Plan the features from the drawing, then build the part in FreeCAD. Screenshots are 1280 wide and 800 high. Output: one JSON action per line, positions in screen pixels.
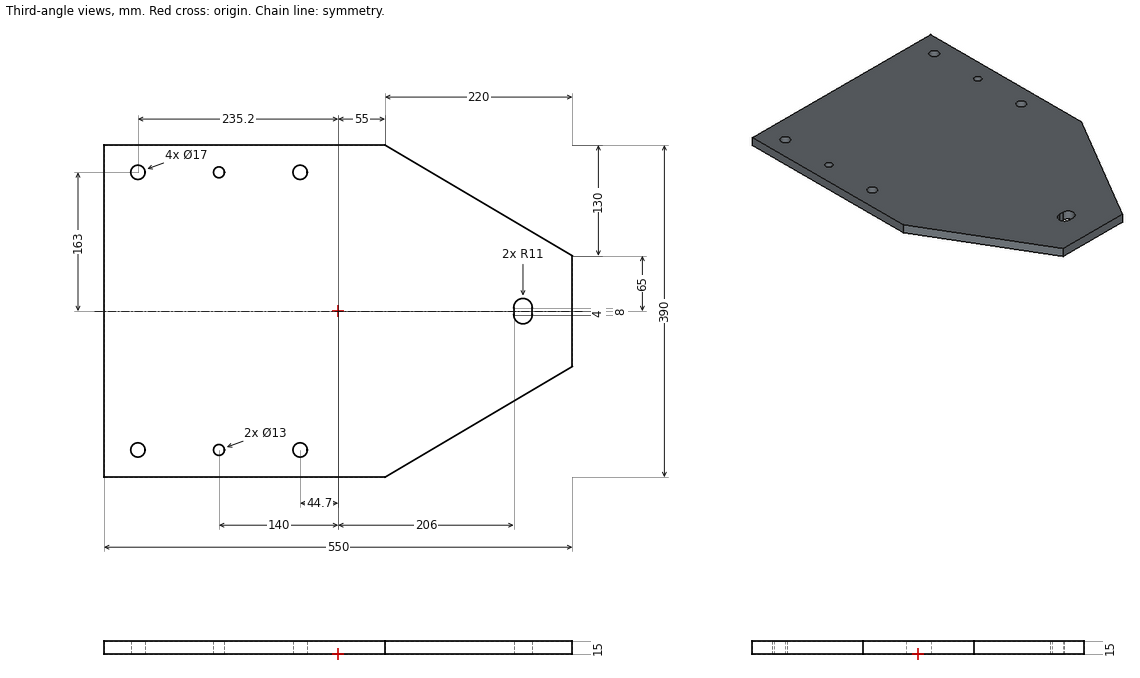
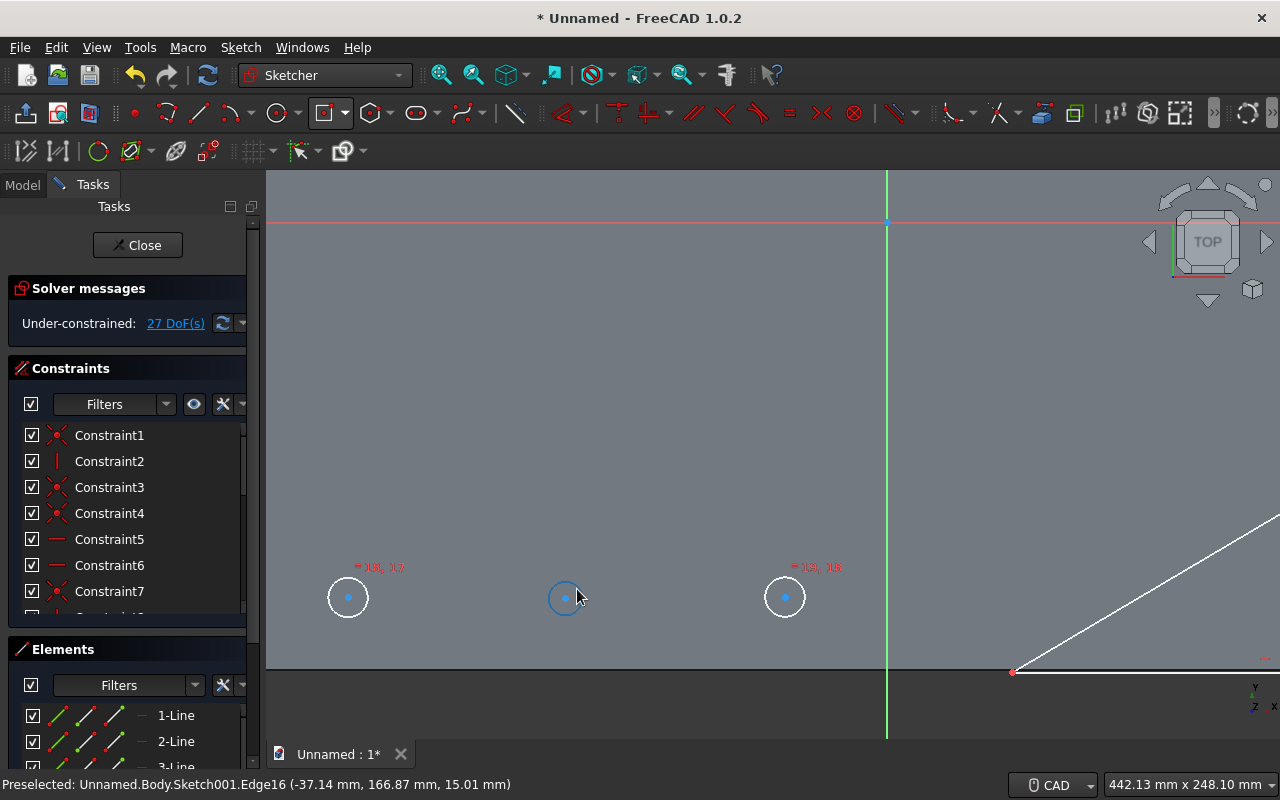
{"action": "left_click", "coordinate": [577, 587]}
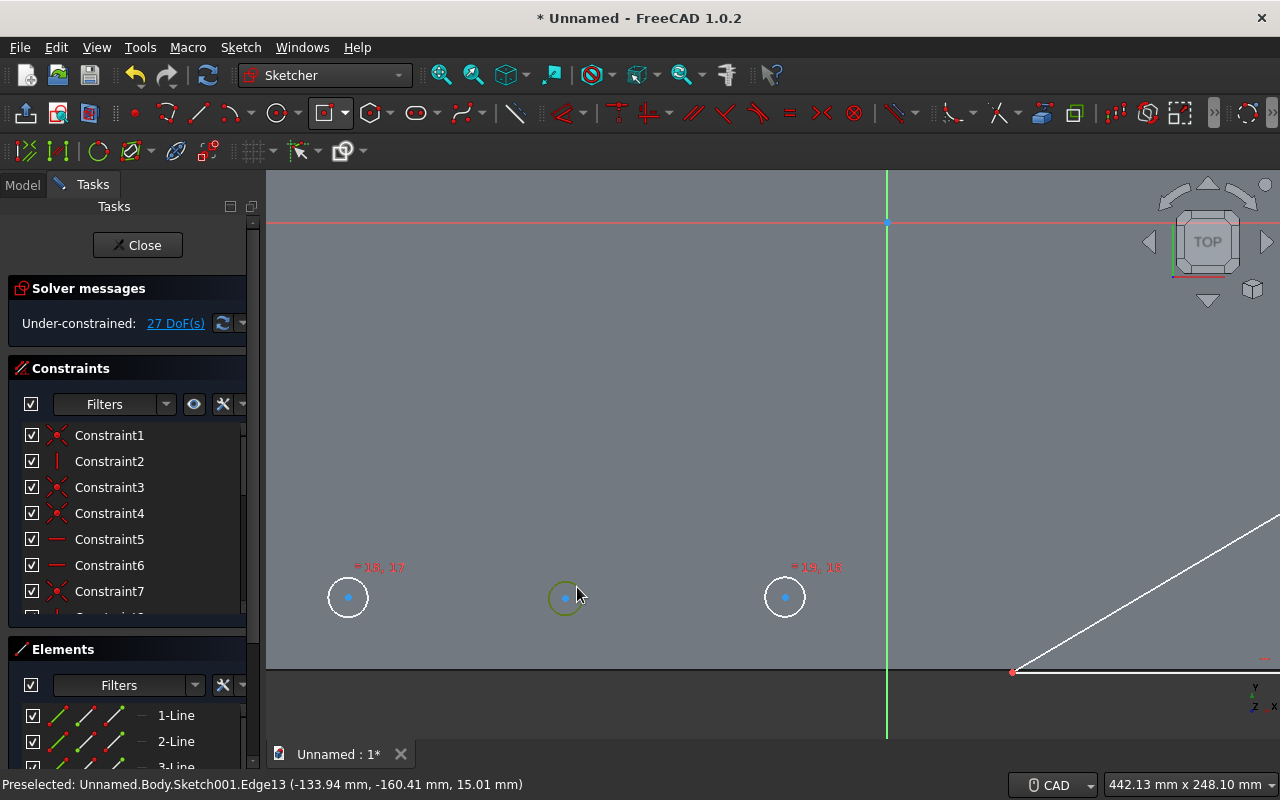
{"action": "scroll", "coordinate": [577, 589], "scroll_direction": "down", "scroll_amount": 5}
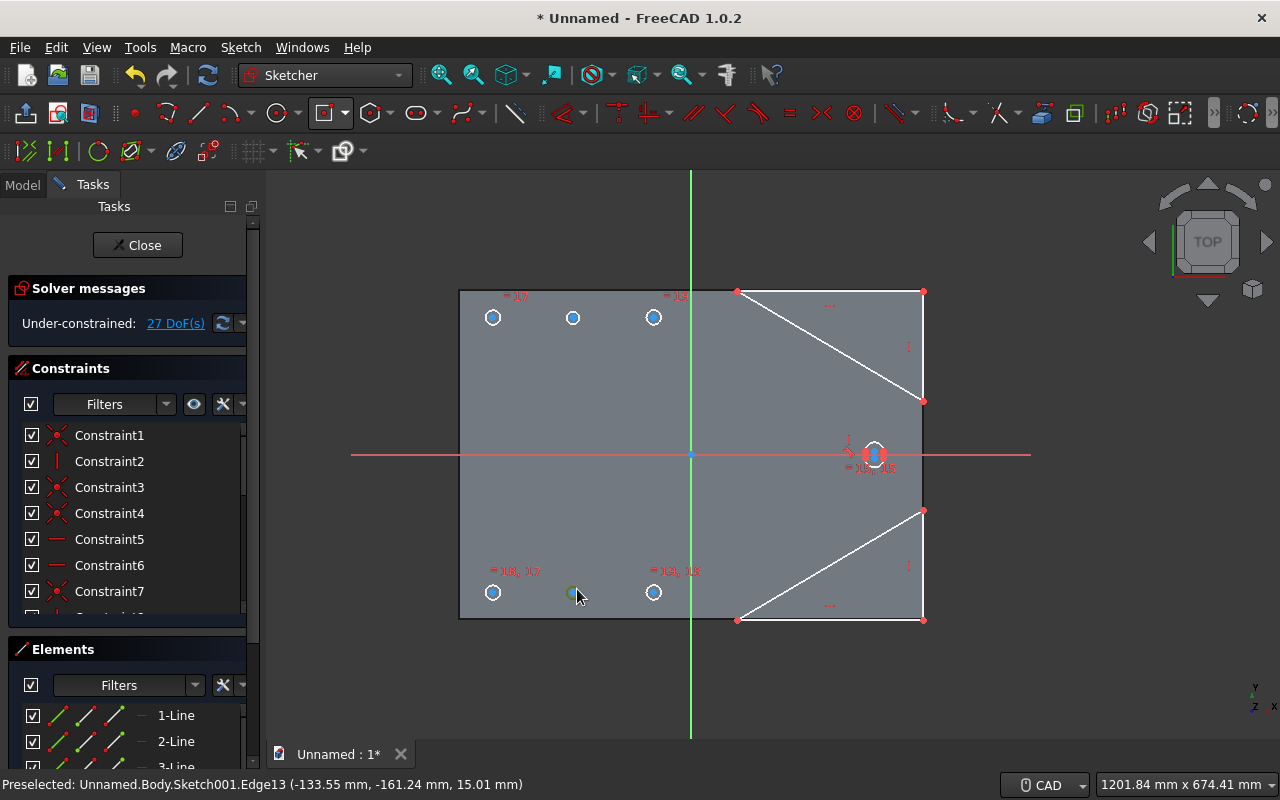
{"action": "scroll", "coordinate": [577, 314], "scroll_direction": "up", "scroll_amount": 5}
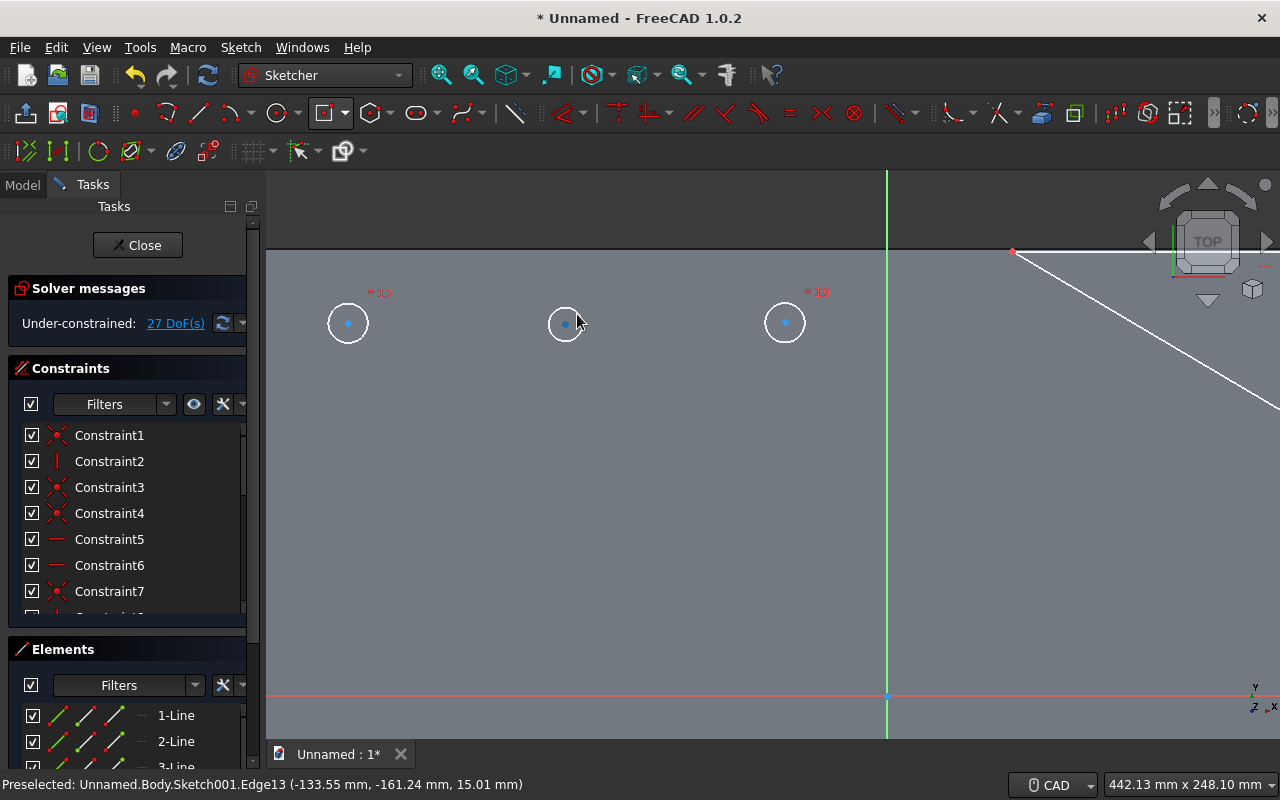
{"action": "left_click", "coordinate": [577, 313]}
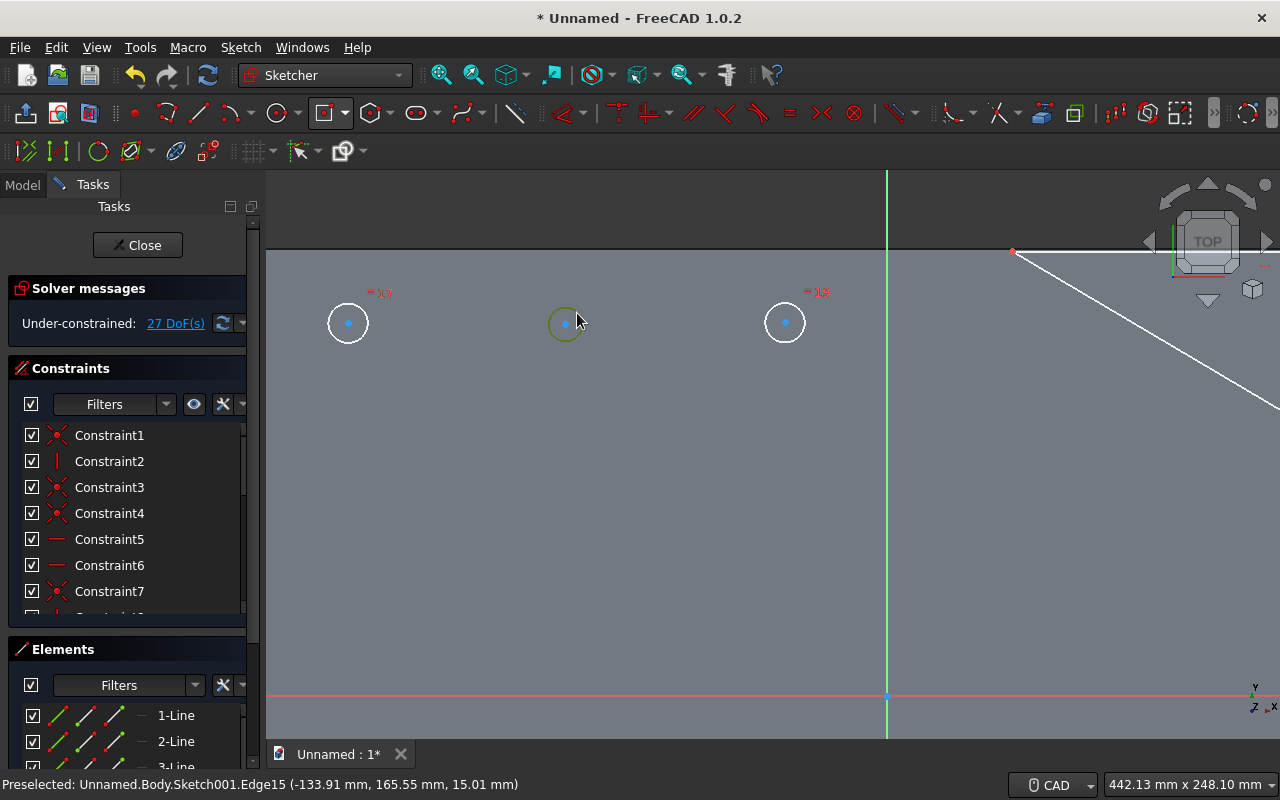
{"action": "left_click", "coordinate": [790, 114]}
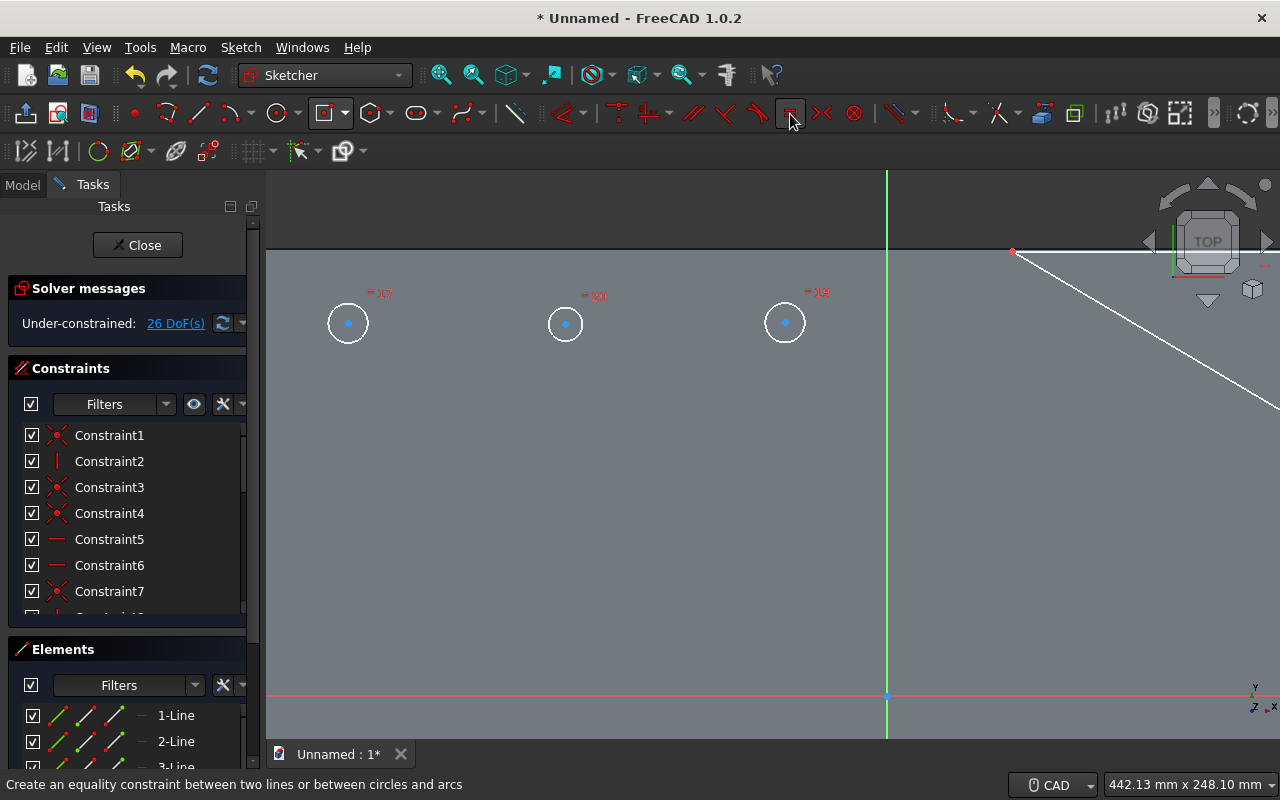
{"action": "left_click", "coordinate": [348, 323]}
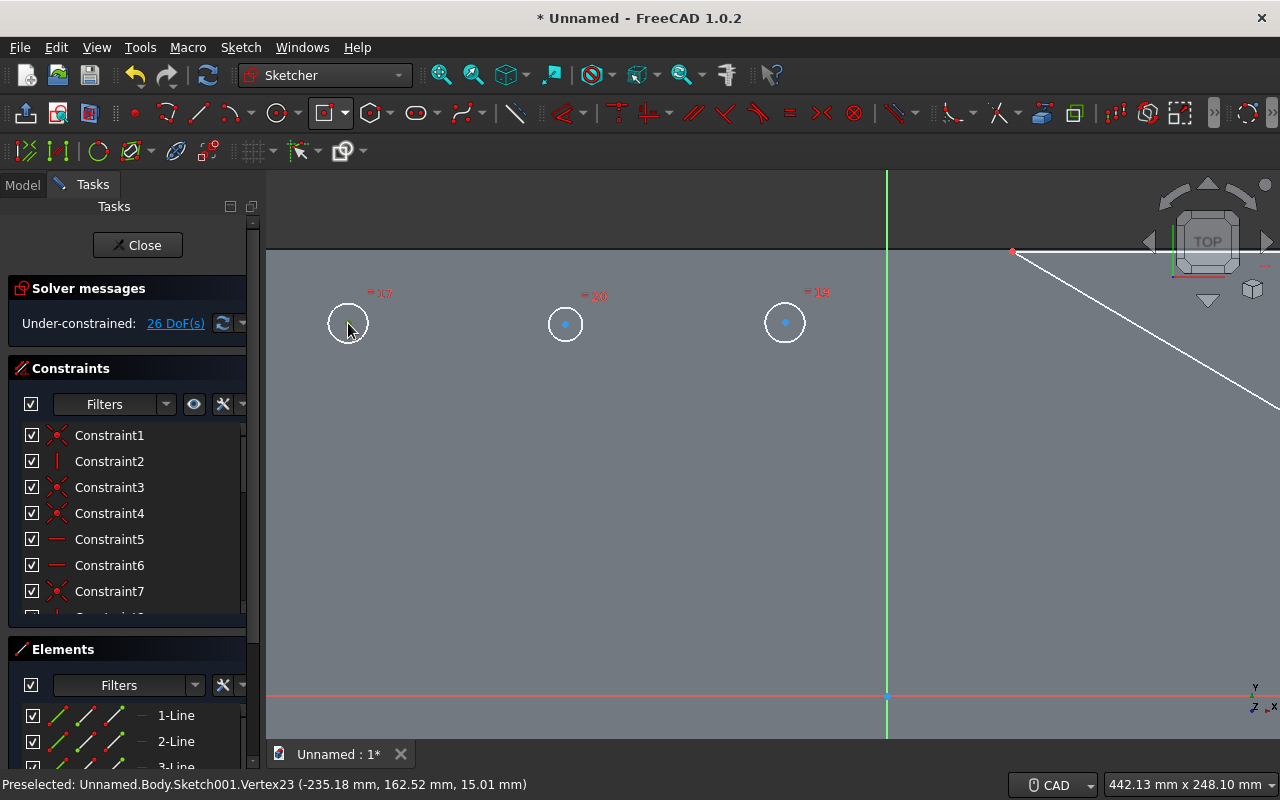
{"action": "scroll", "coordinate": [577, 314], "scroll_direction": "down", "scroll_amount": 5}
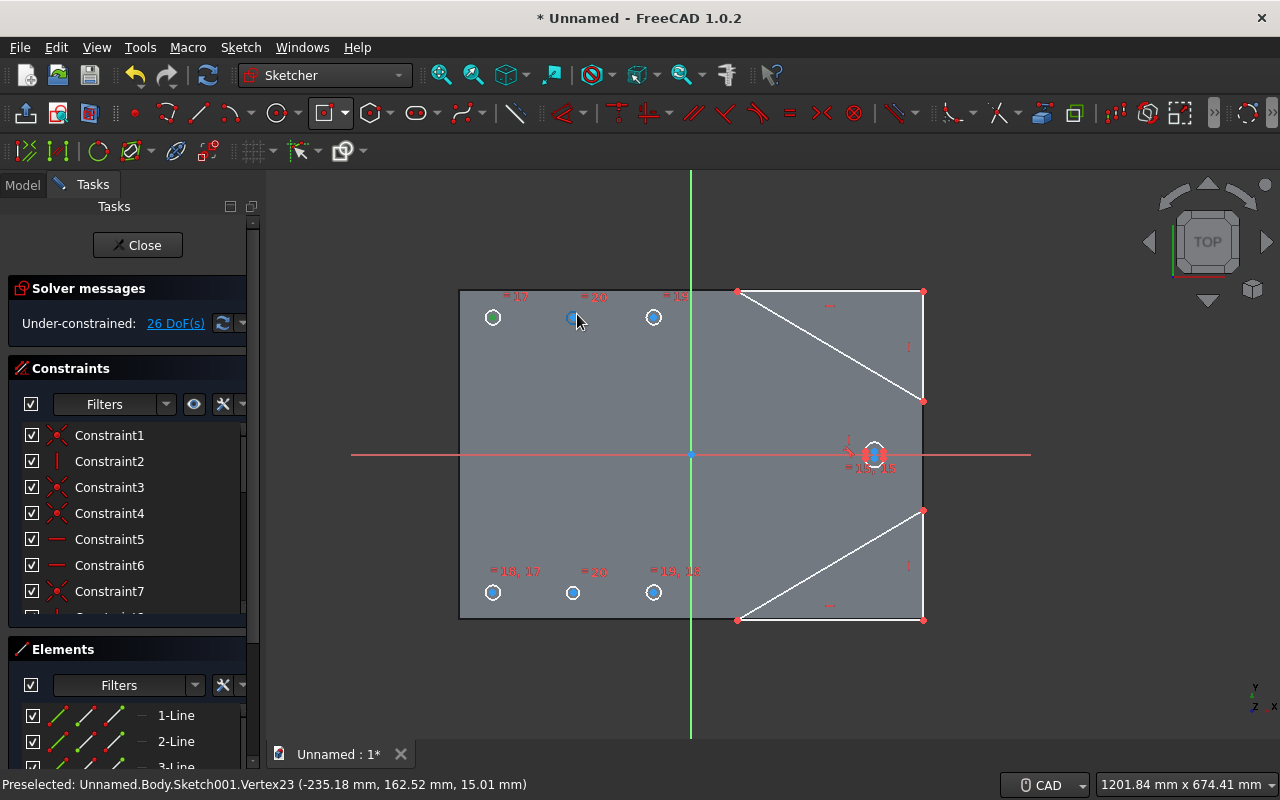
{"action": "left_click", "coordinate": [493, 593]}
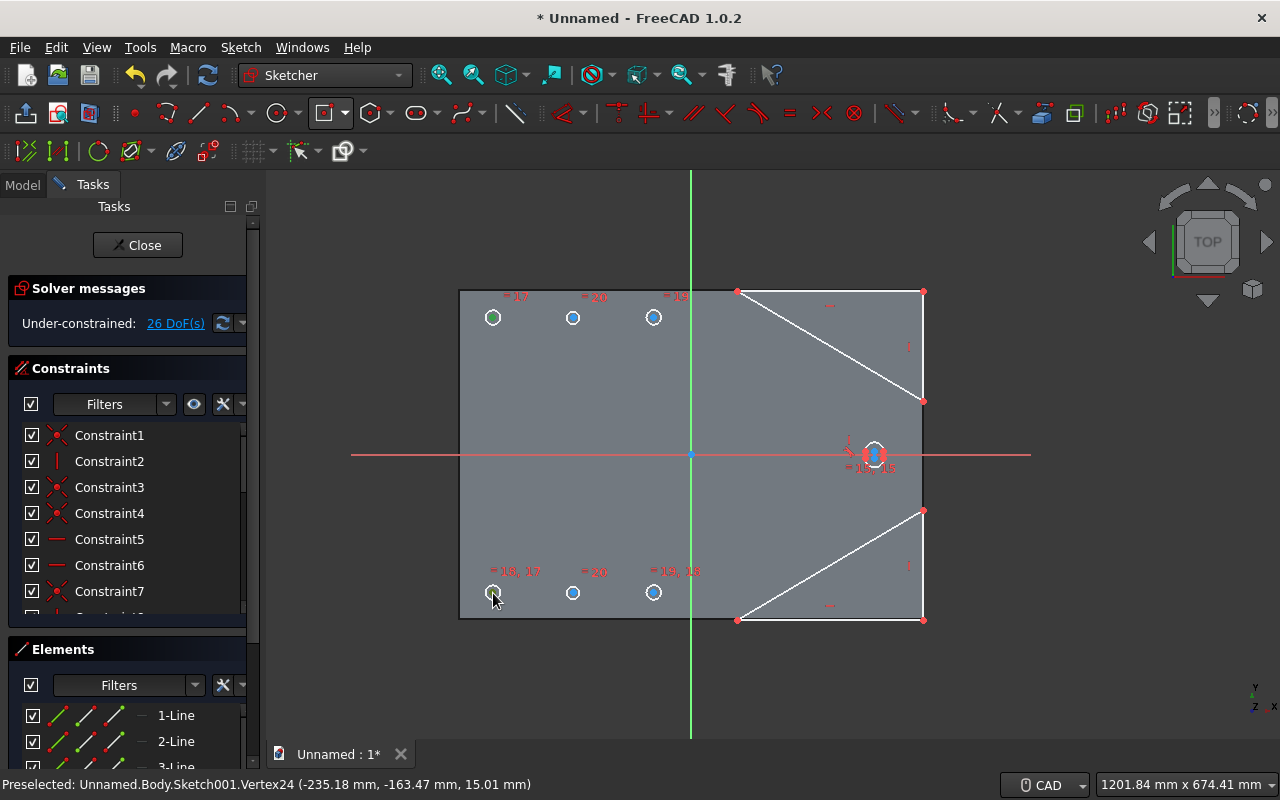
{"action": "left_click", "coordinate": [672, 114]}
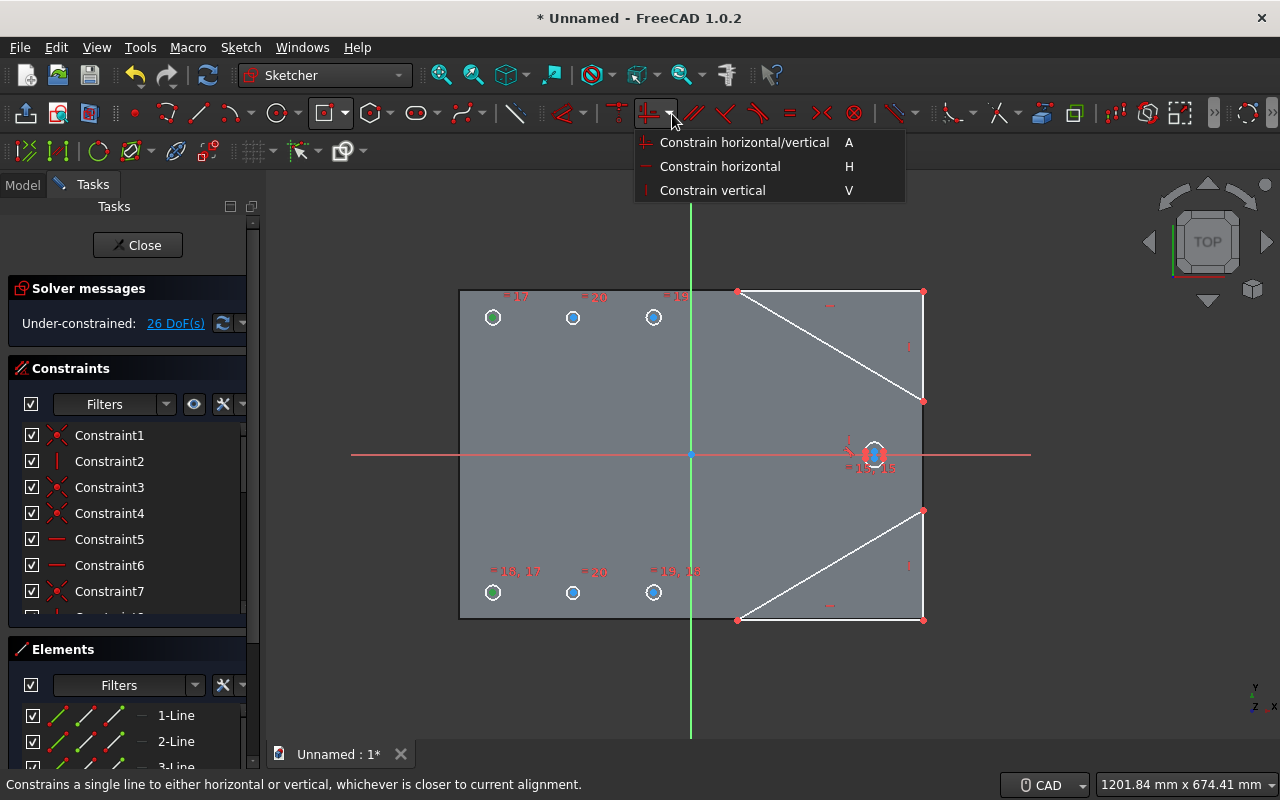
{"action": "left_click", "coordinate": [770, 190]}